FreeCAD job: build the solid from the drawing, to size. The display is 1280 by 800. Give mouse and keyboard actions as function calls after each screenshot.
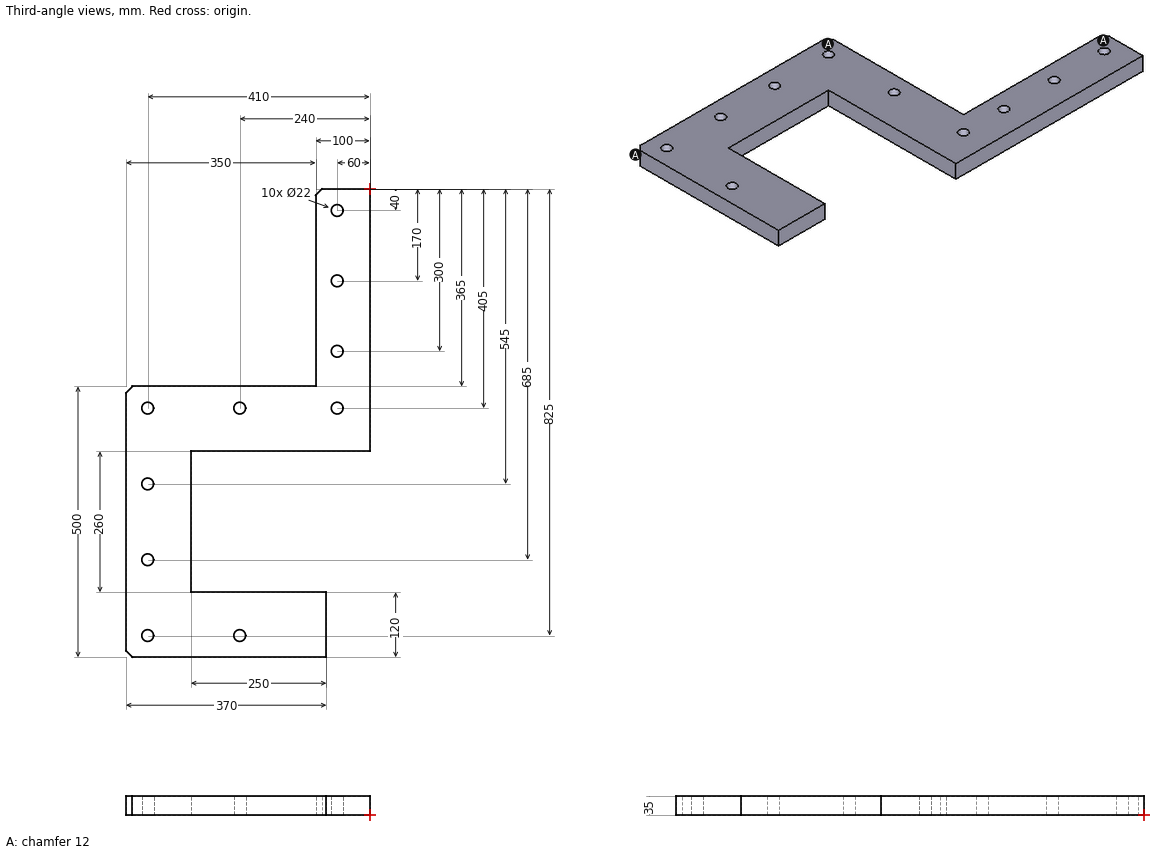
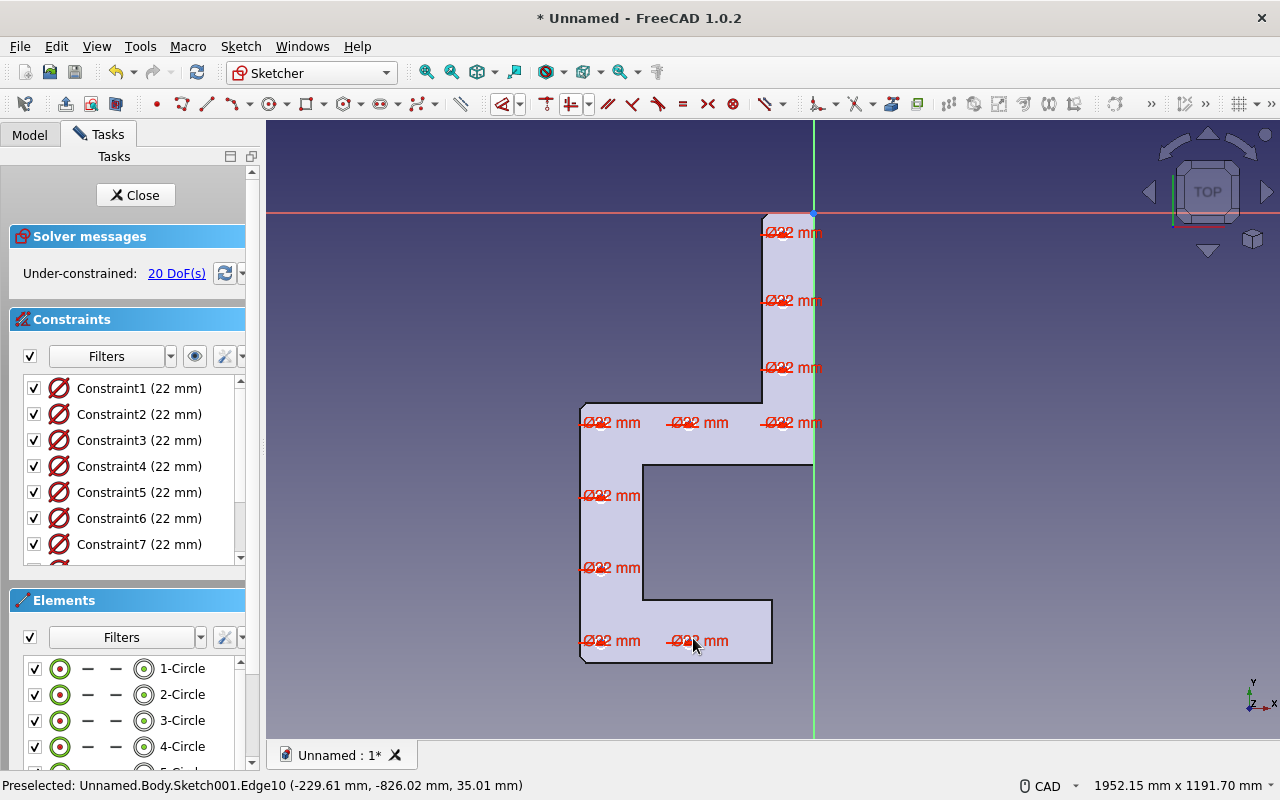
click(783, 235)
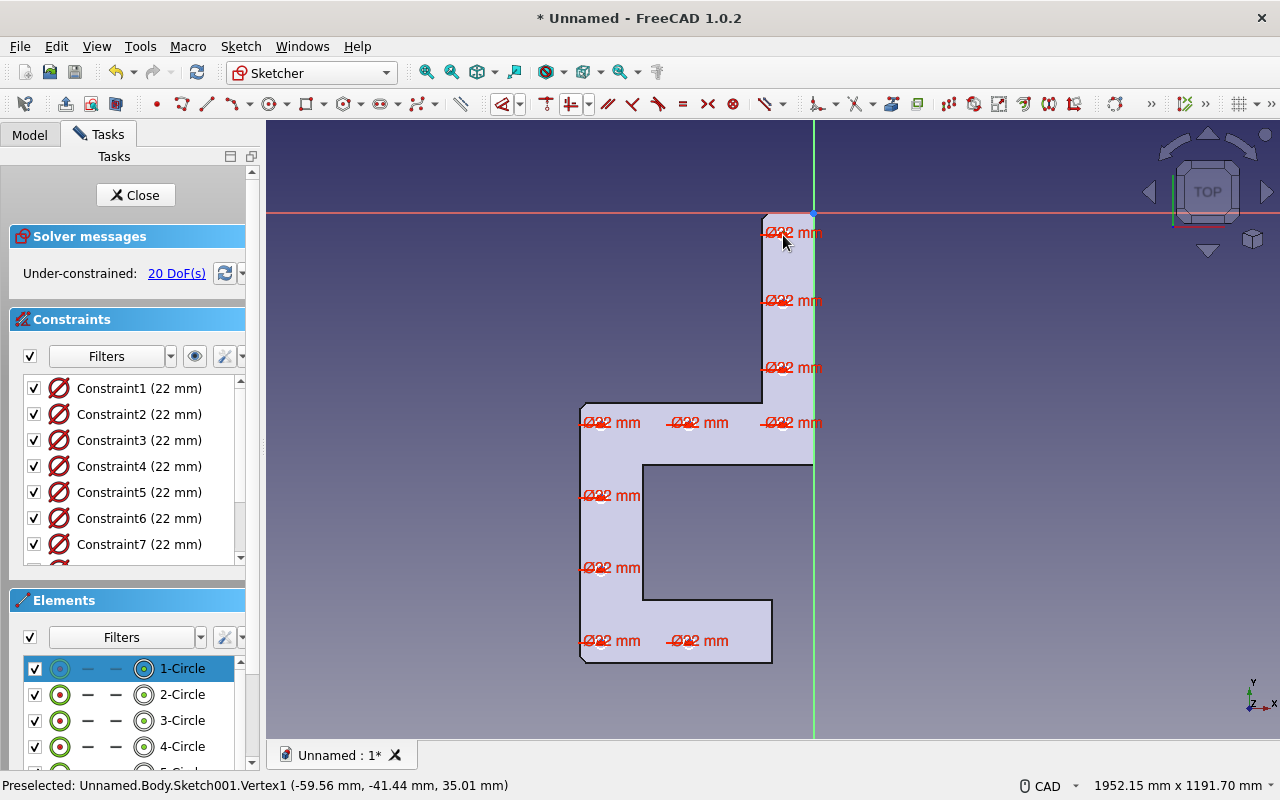
click(783, 303)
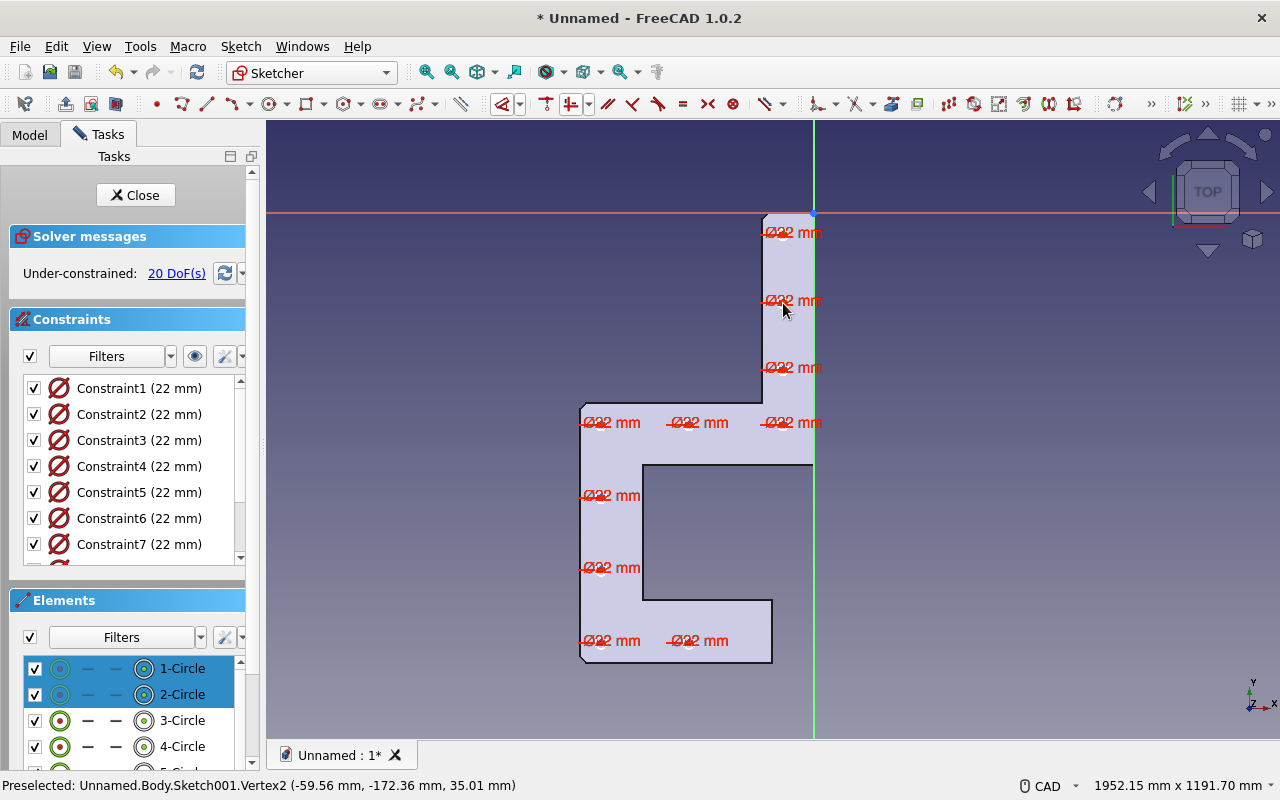
click(588, 104)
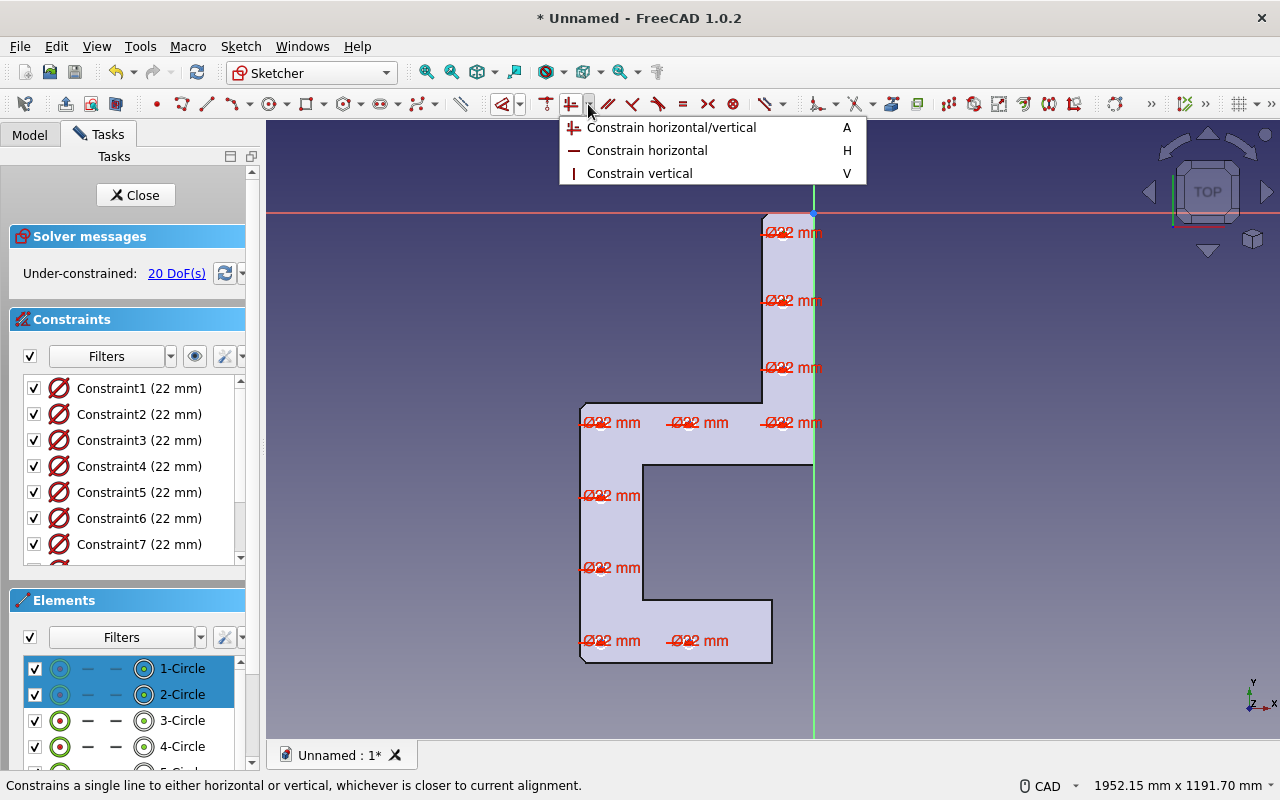
click(713, 174)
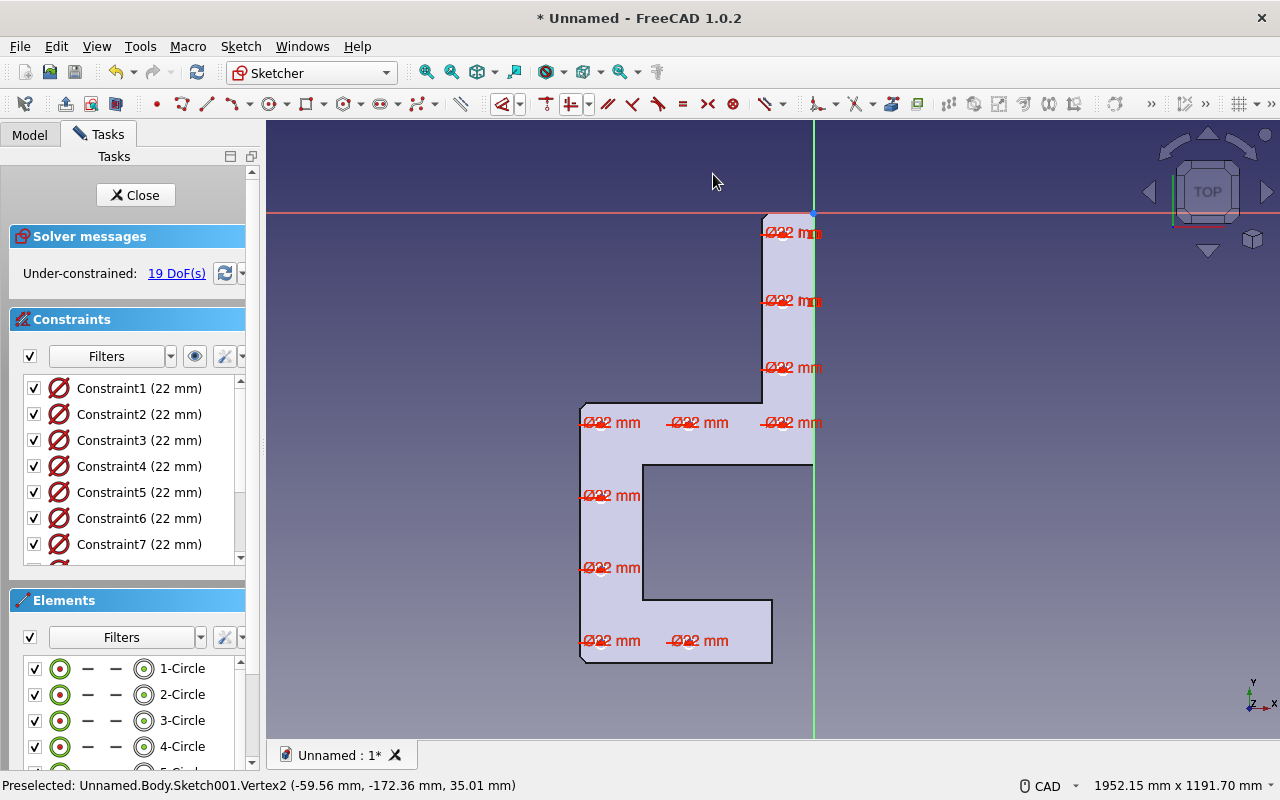
click(783, 303)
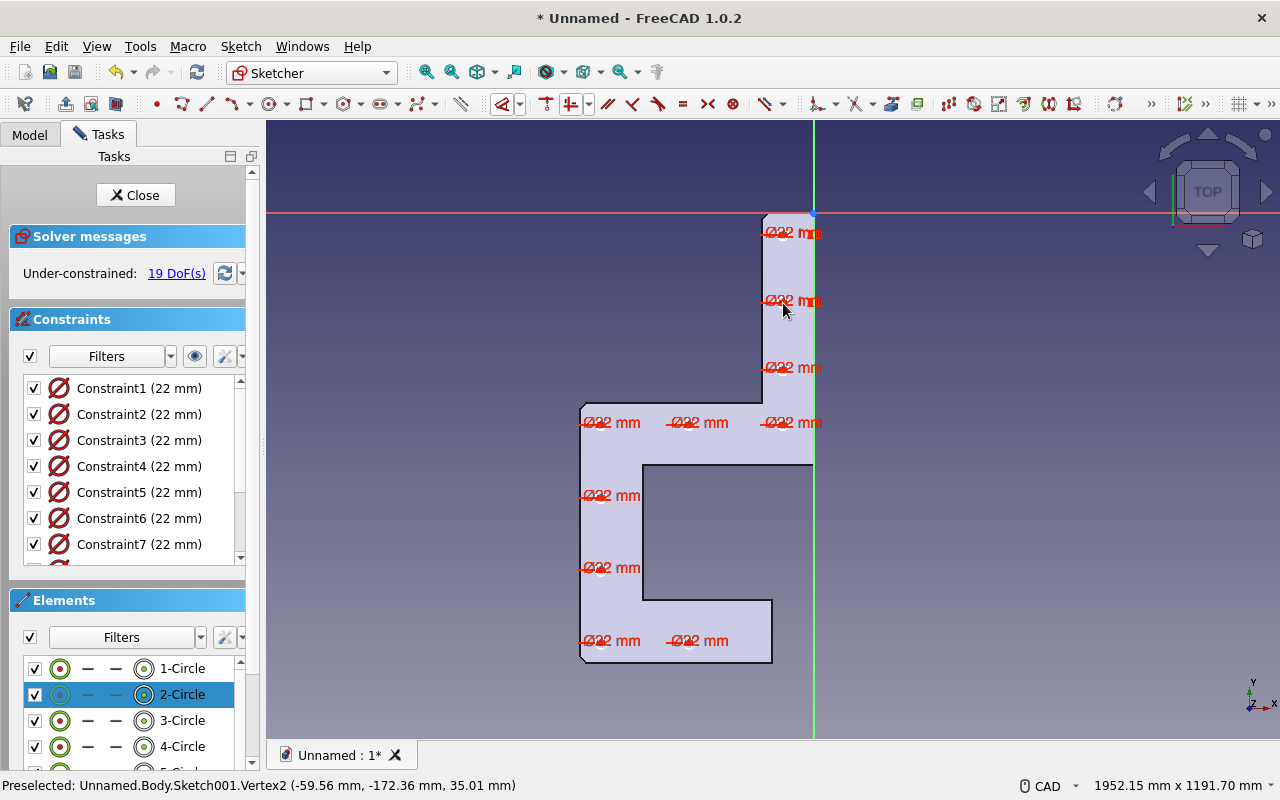
click(783, 370)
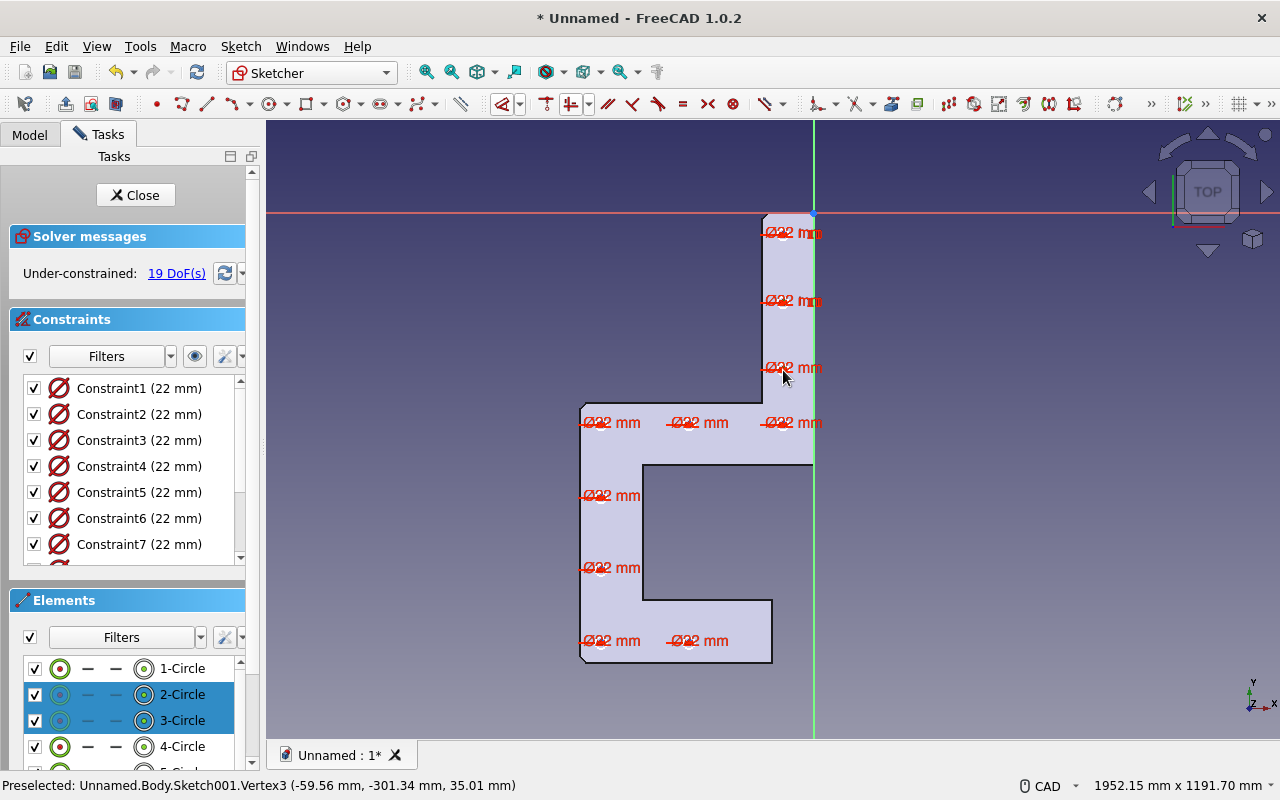
key(v)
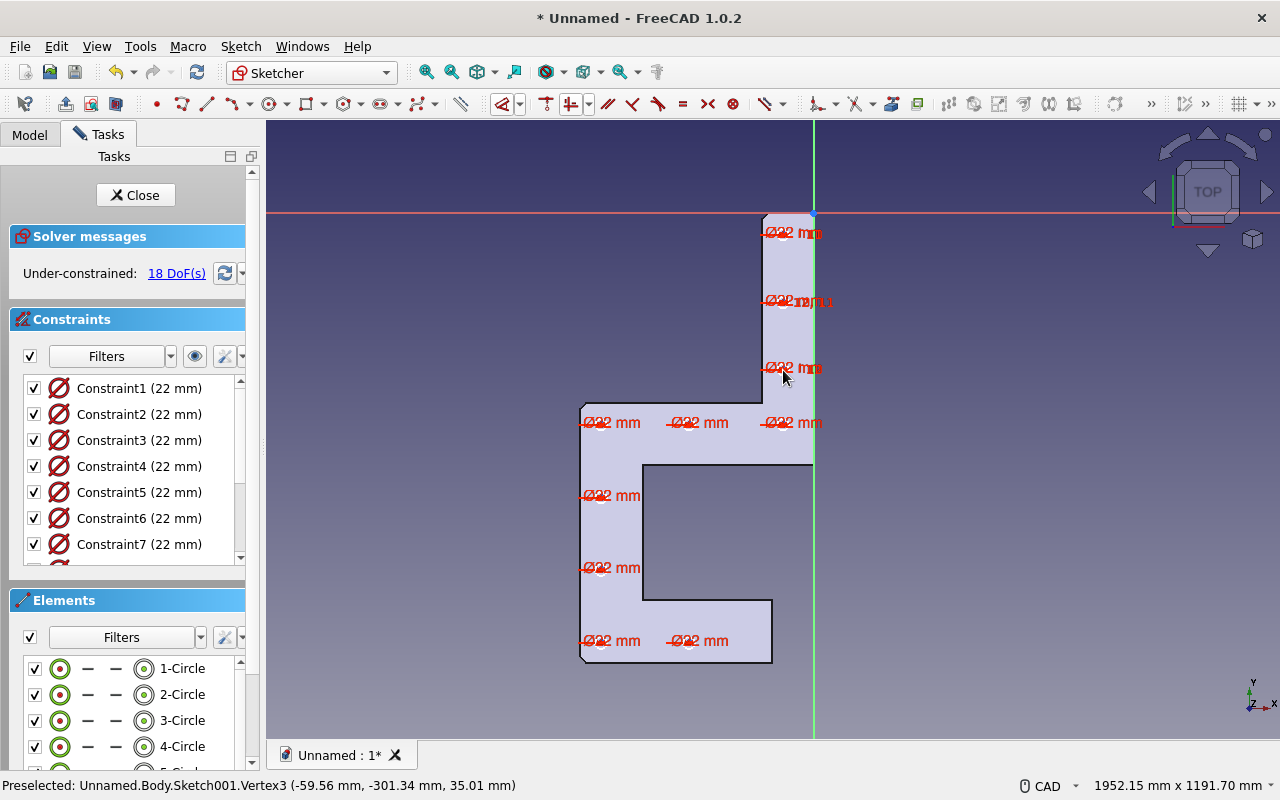
click(783, 370)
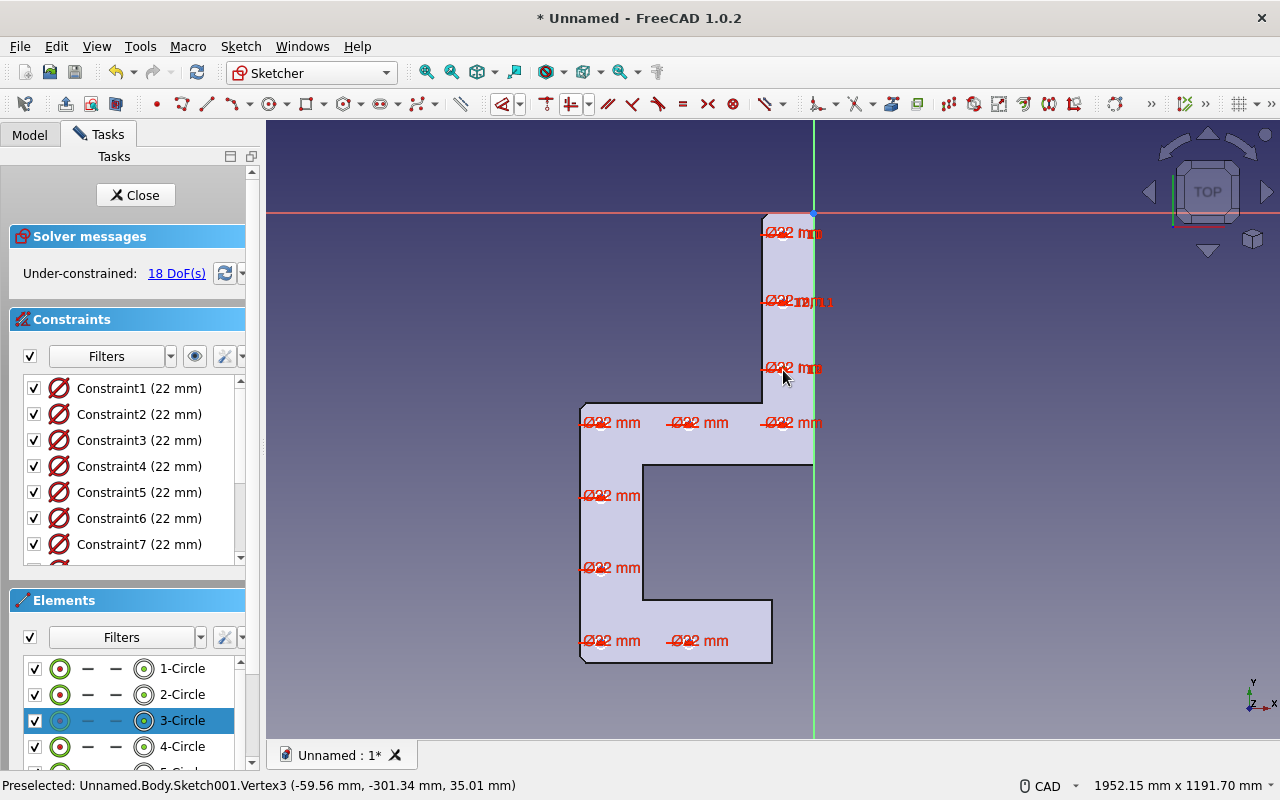
click(783, 425)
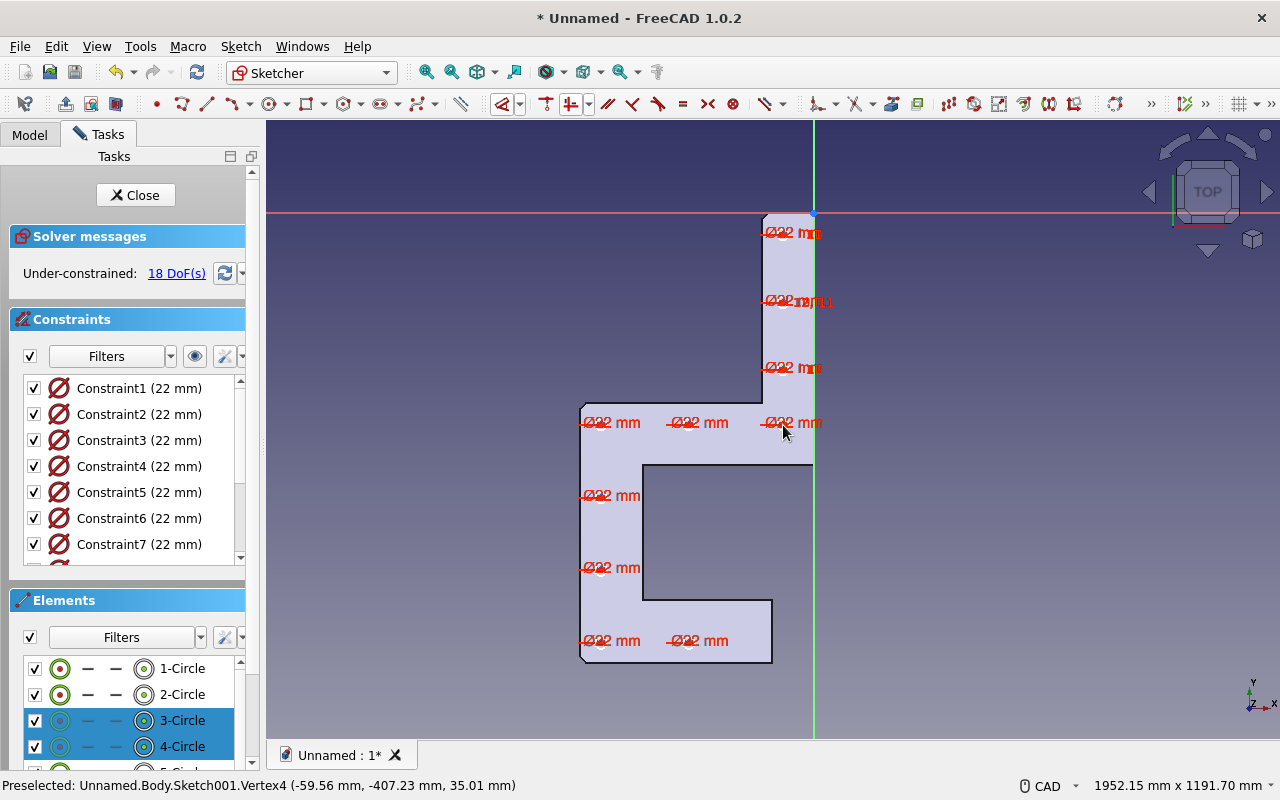
click(588, 104)